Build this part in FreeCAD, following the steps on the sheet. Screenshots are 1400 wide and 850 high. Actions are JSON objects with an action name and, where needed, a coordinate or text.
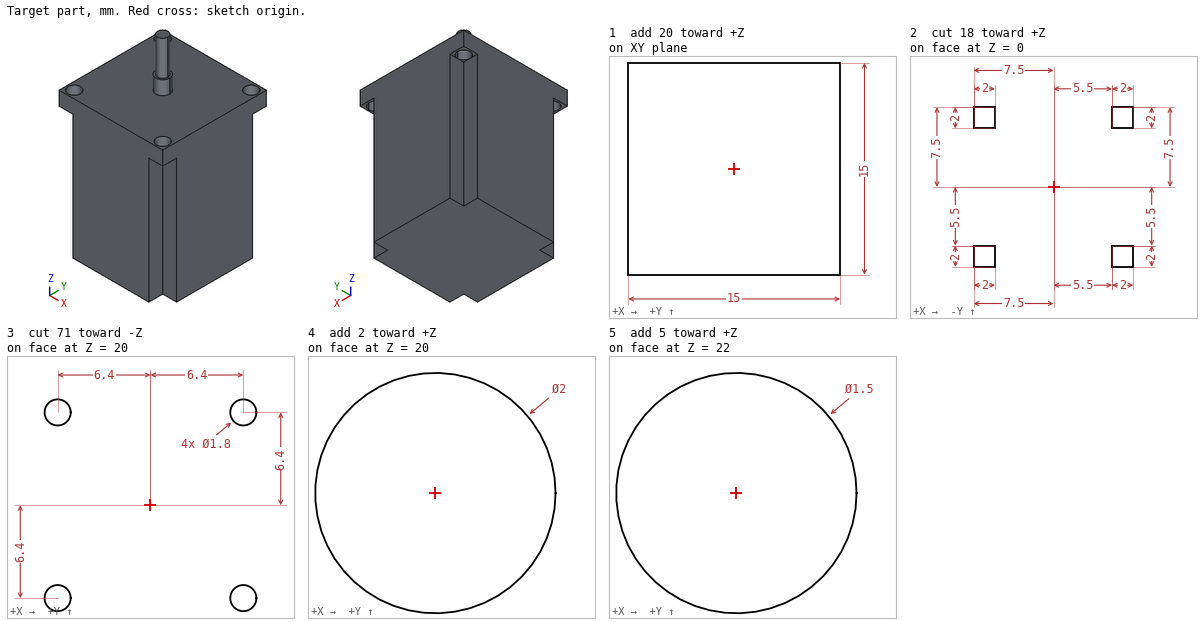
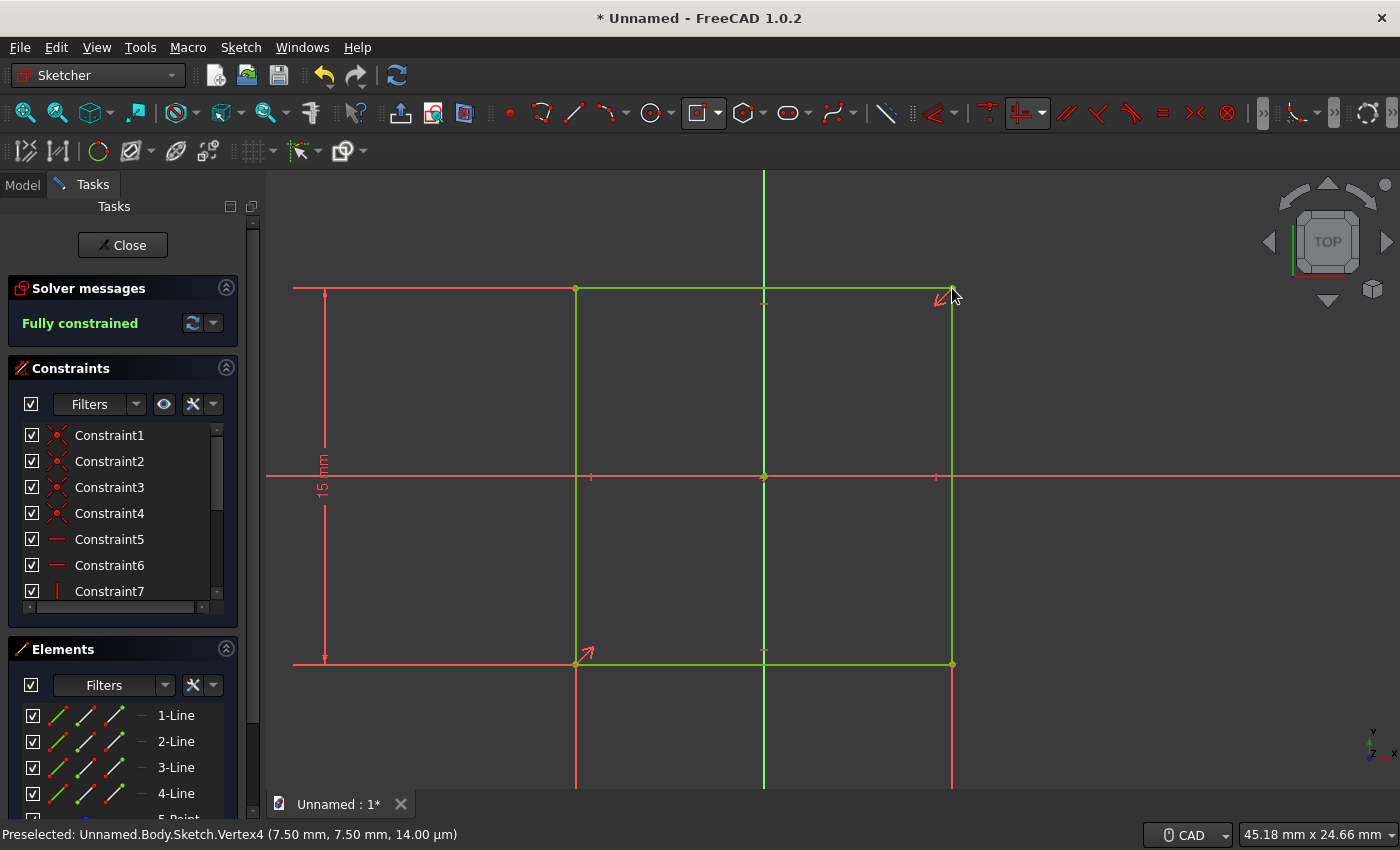
{"action": "left_click", "coordinate": [123, 245]}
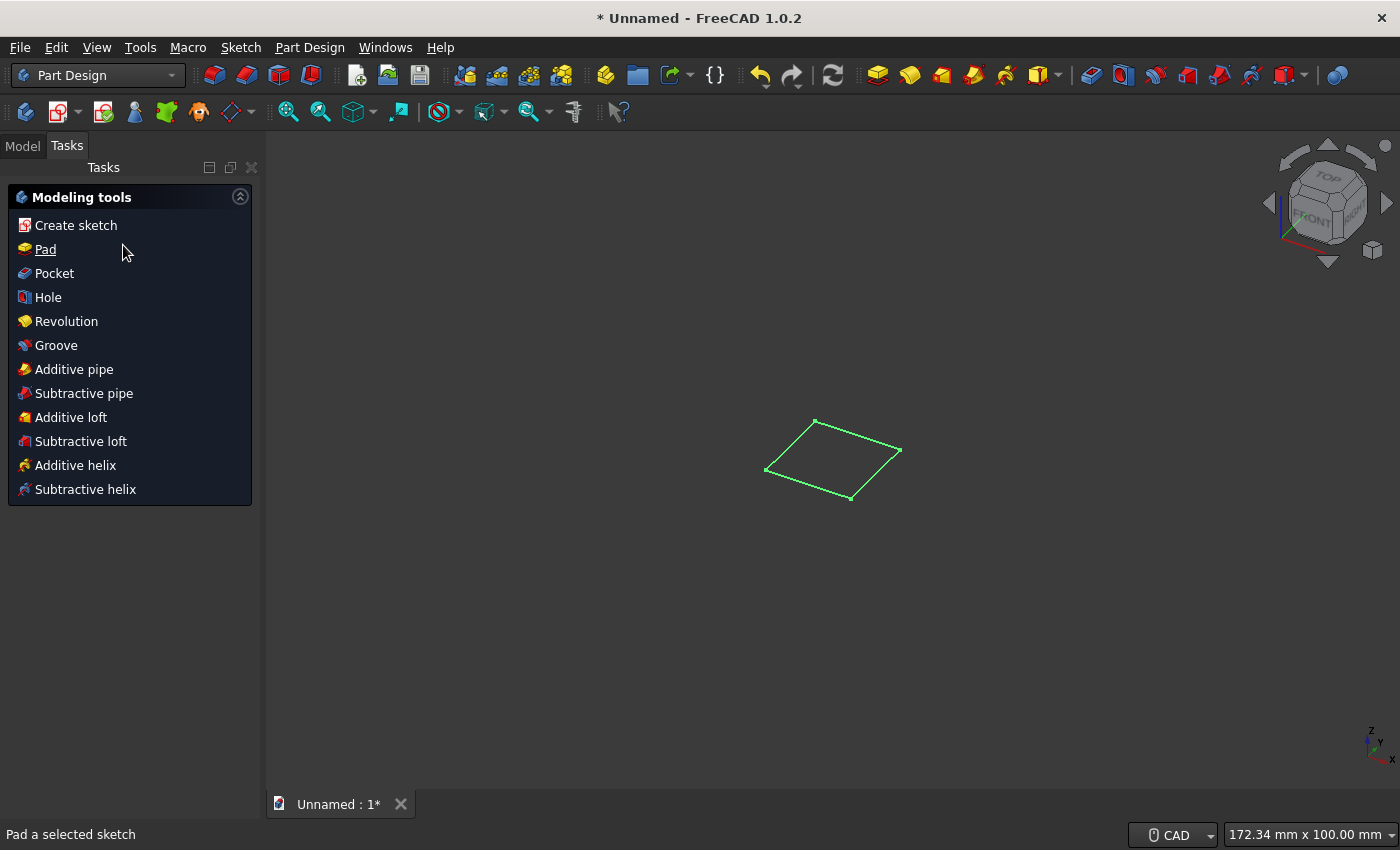
{"action": "left_click", "coordinate": [878, 76]}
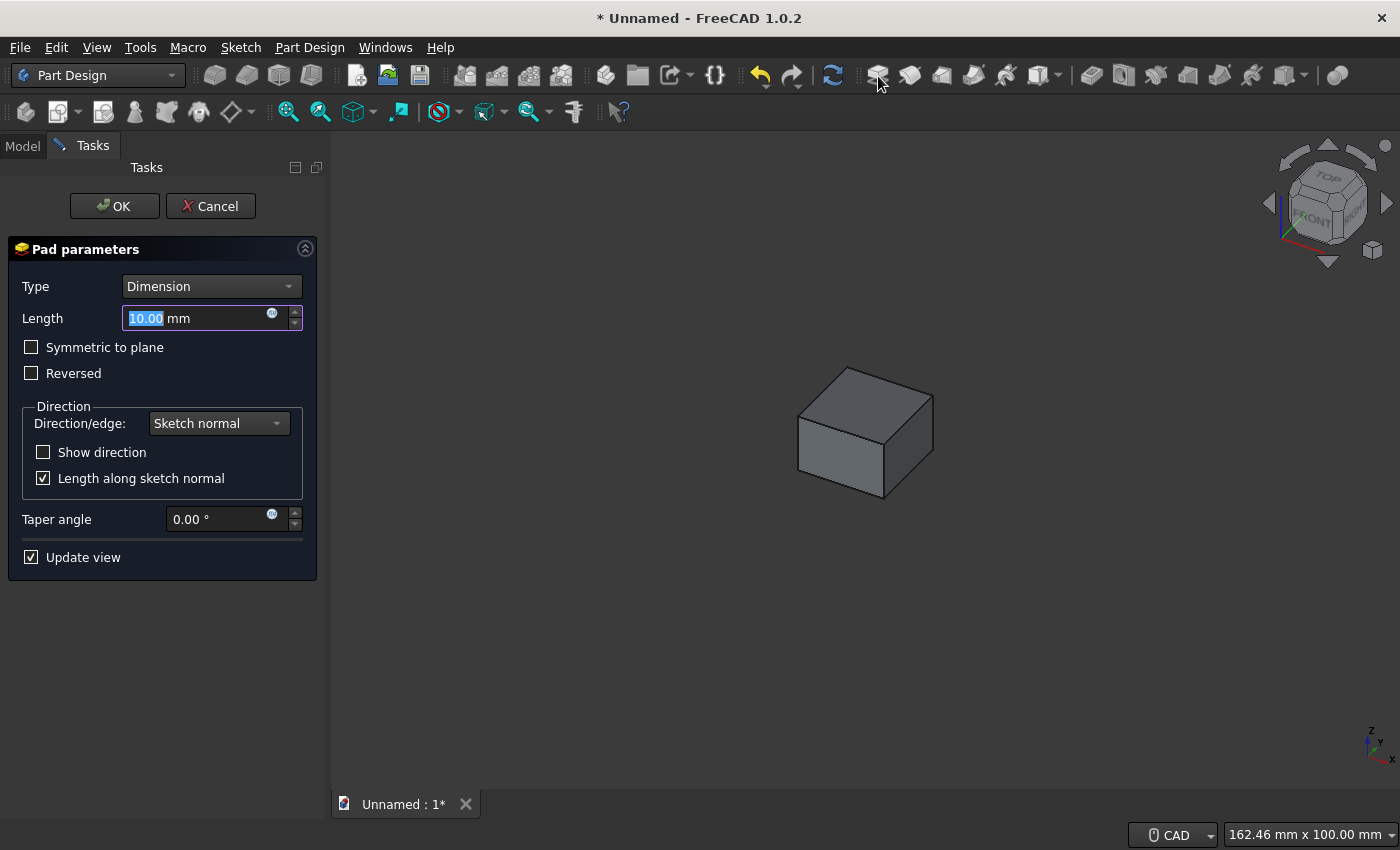
{"action": "type", "text": "20"}
{"action": "key", "text": "Tab"}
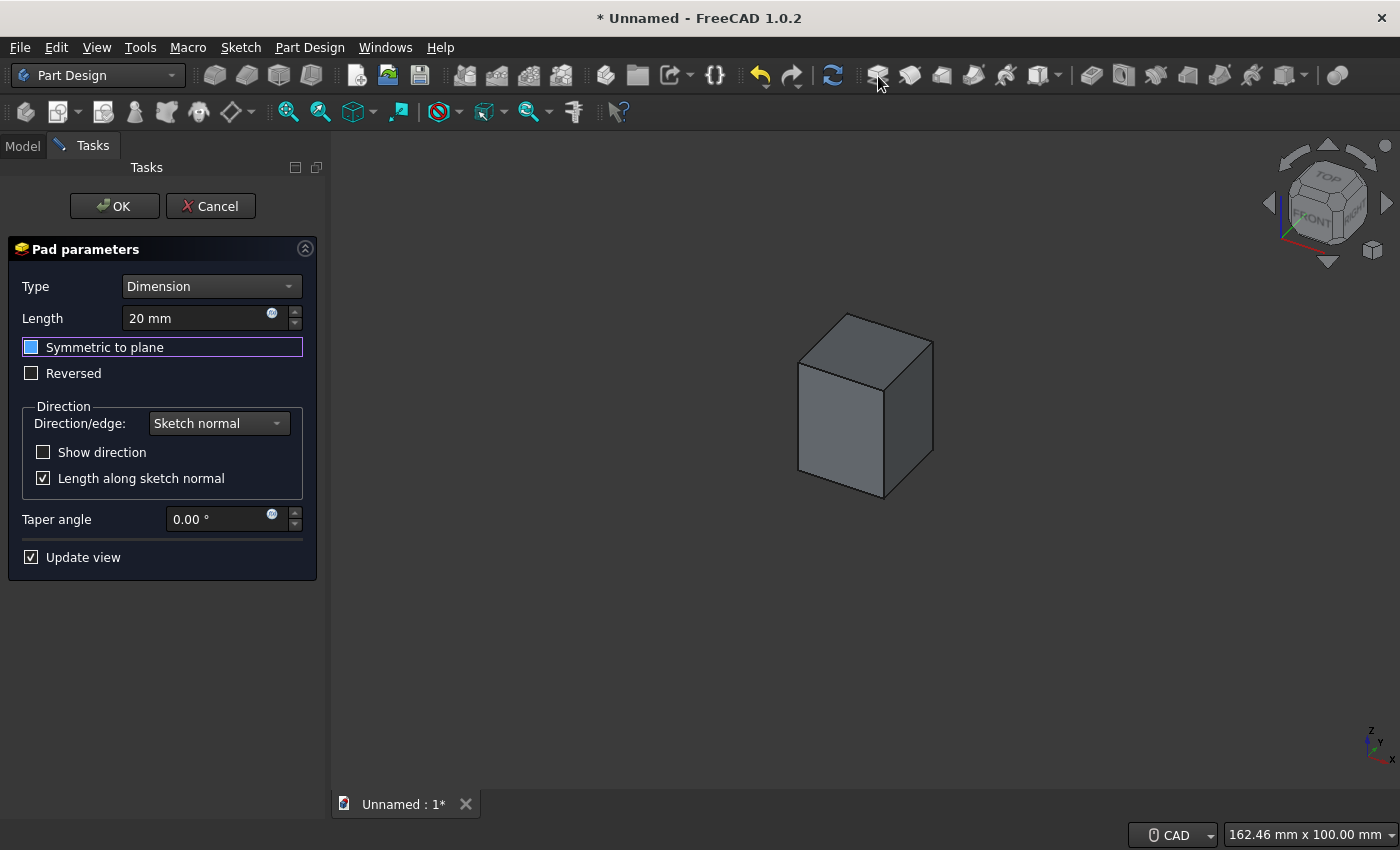
{"action": "left_click", "coordinate": [115, 206]}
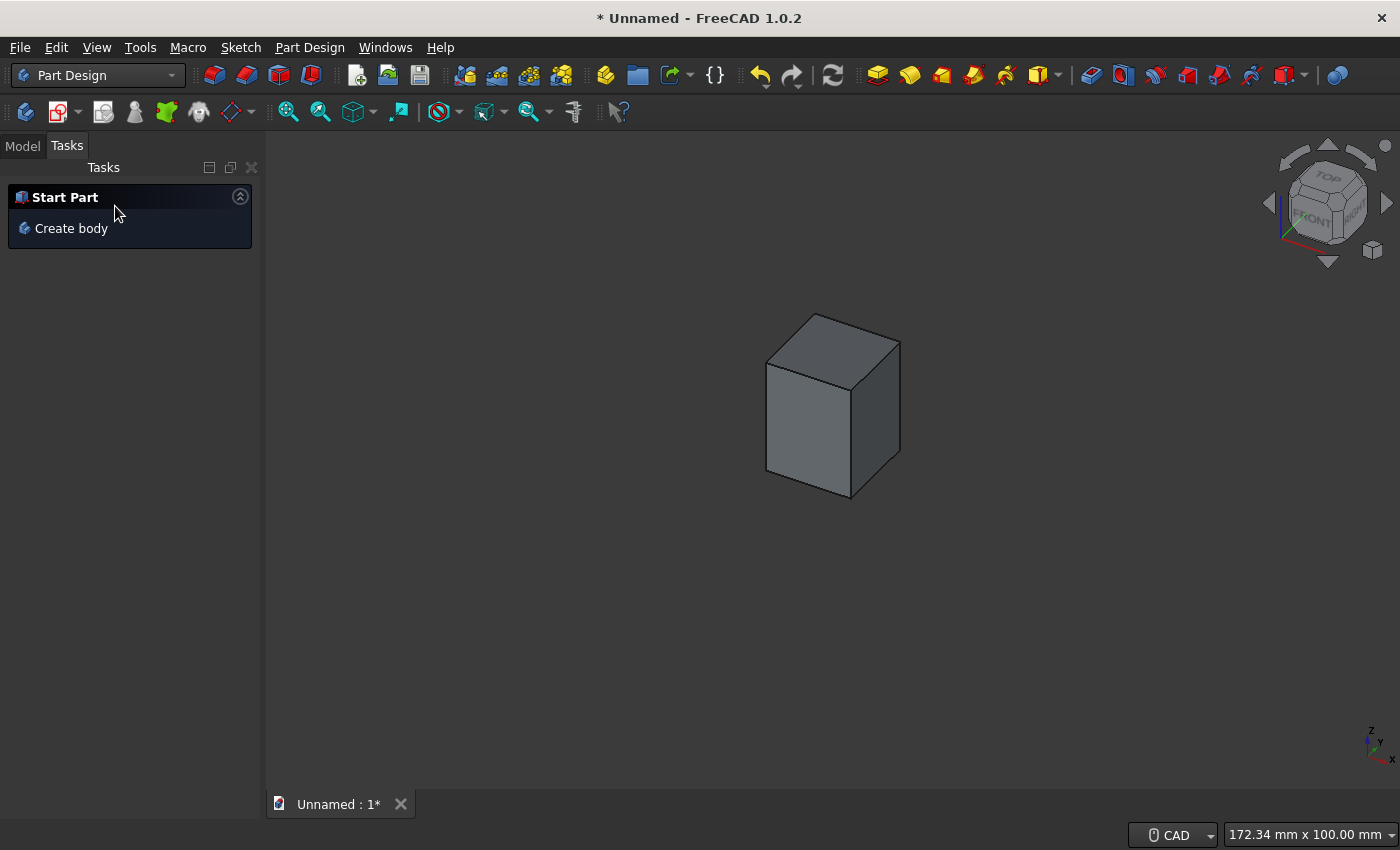
{"action": "left_click", "coordinate": [290, 112]}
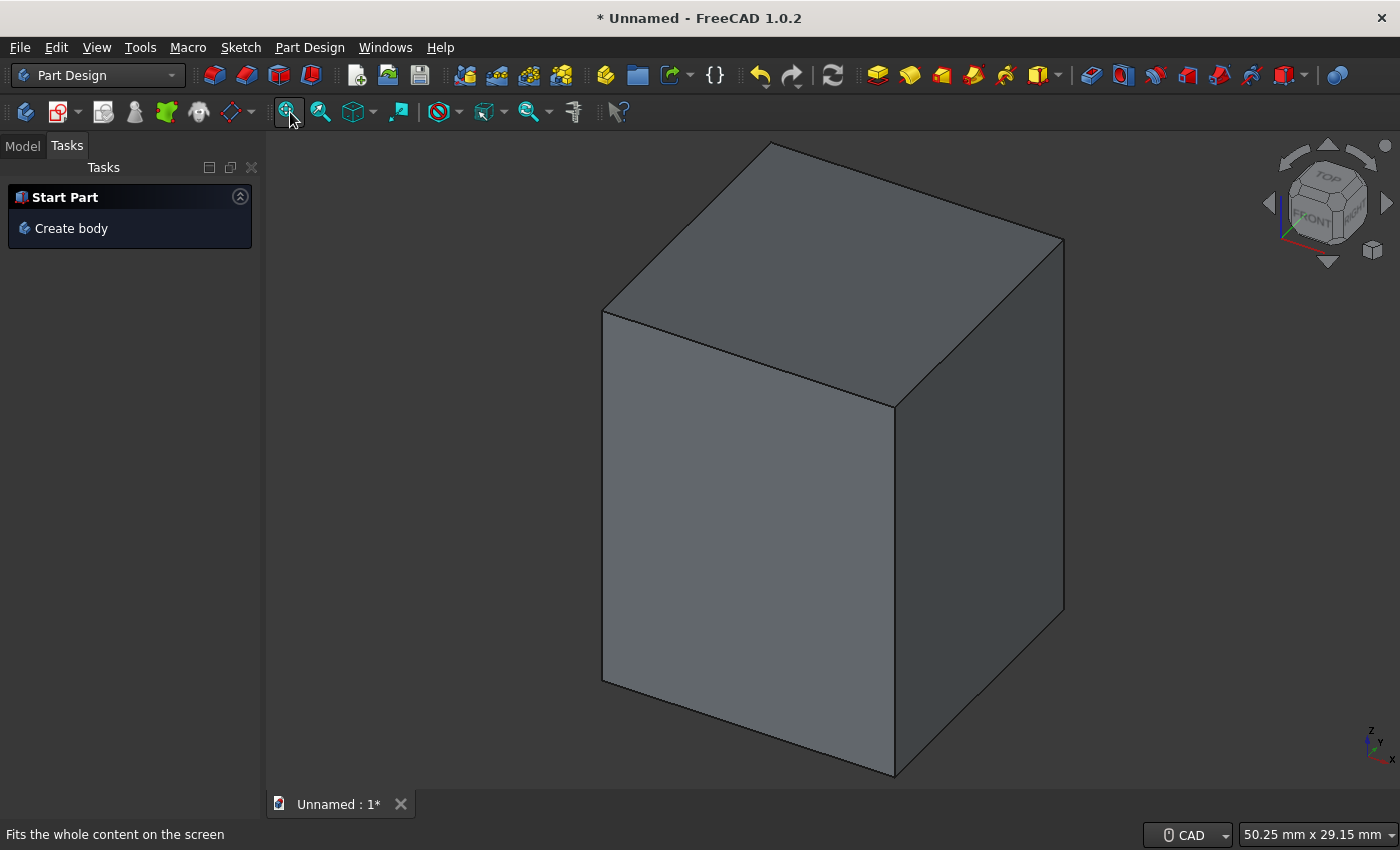
{"action": "key", "text": "5"}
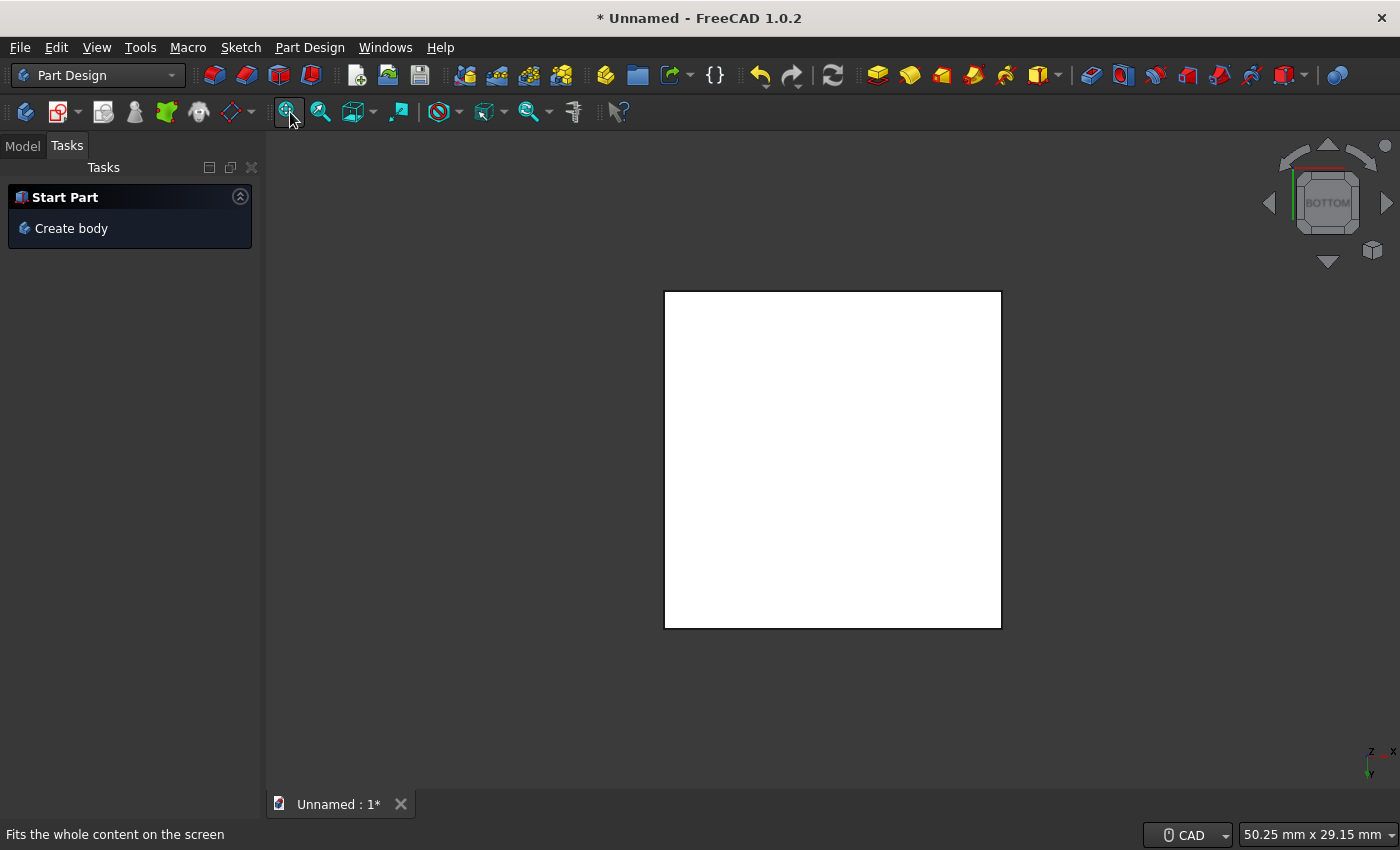
{"action": "left_click", "coordinate": [833, 459]}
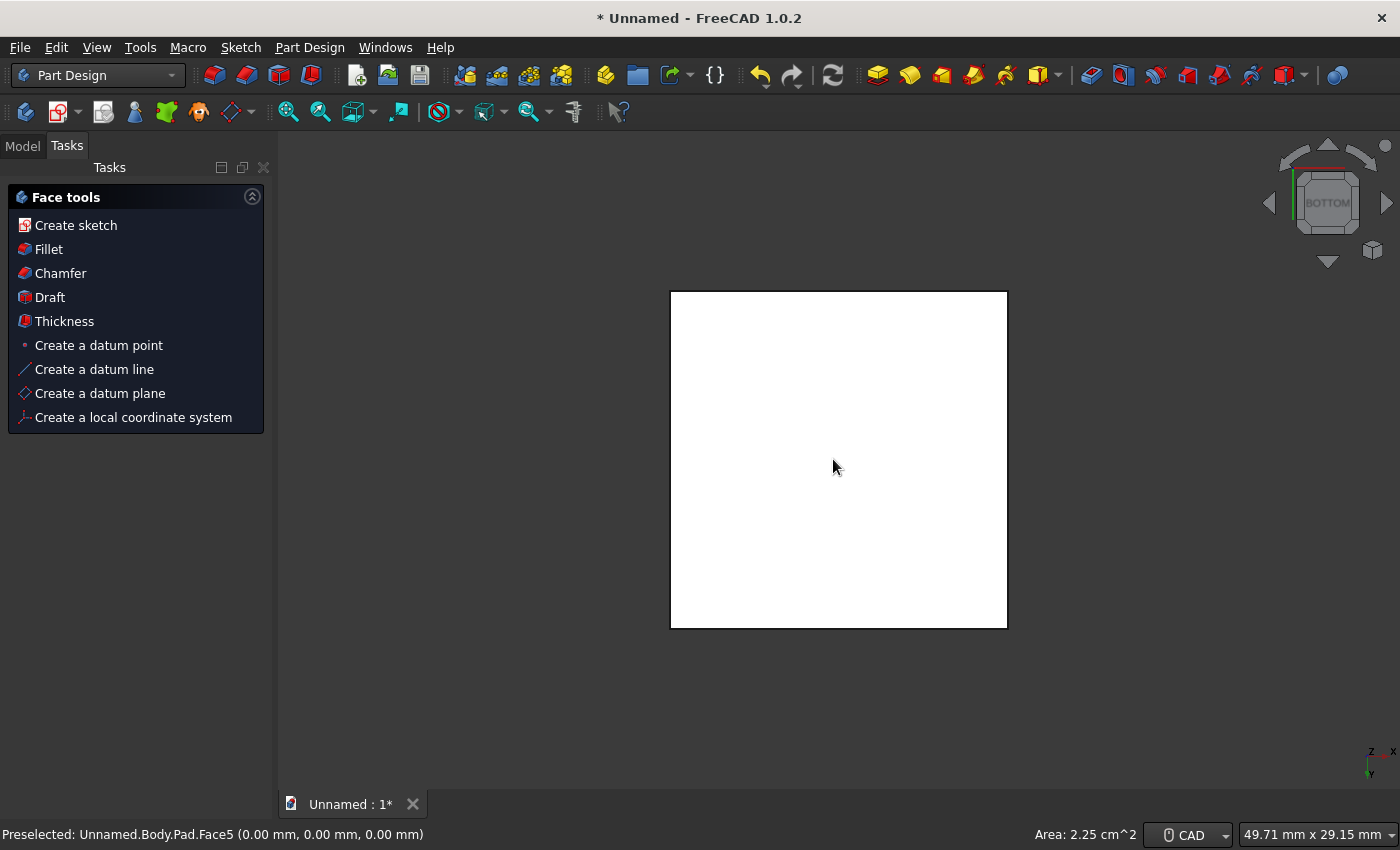
{"action": "left_click", "coordinate": [58, 112]}